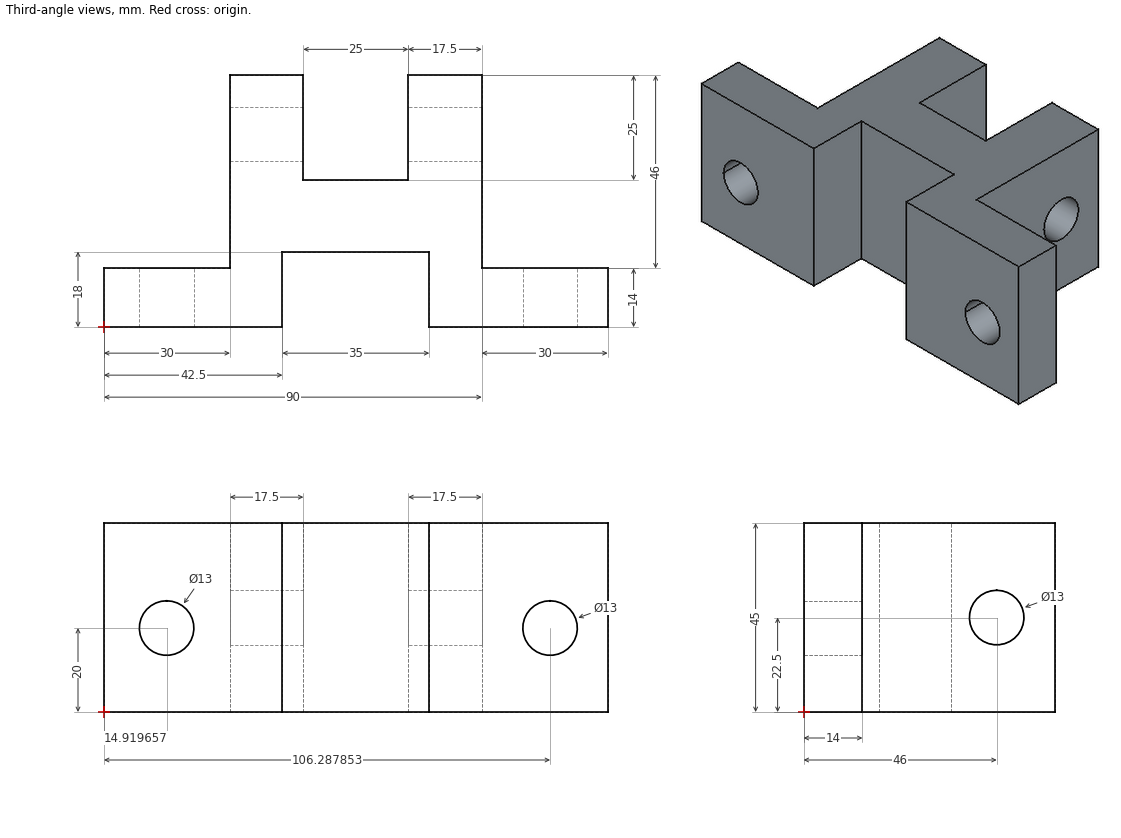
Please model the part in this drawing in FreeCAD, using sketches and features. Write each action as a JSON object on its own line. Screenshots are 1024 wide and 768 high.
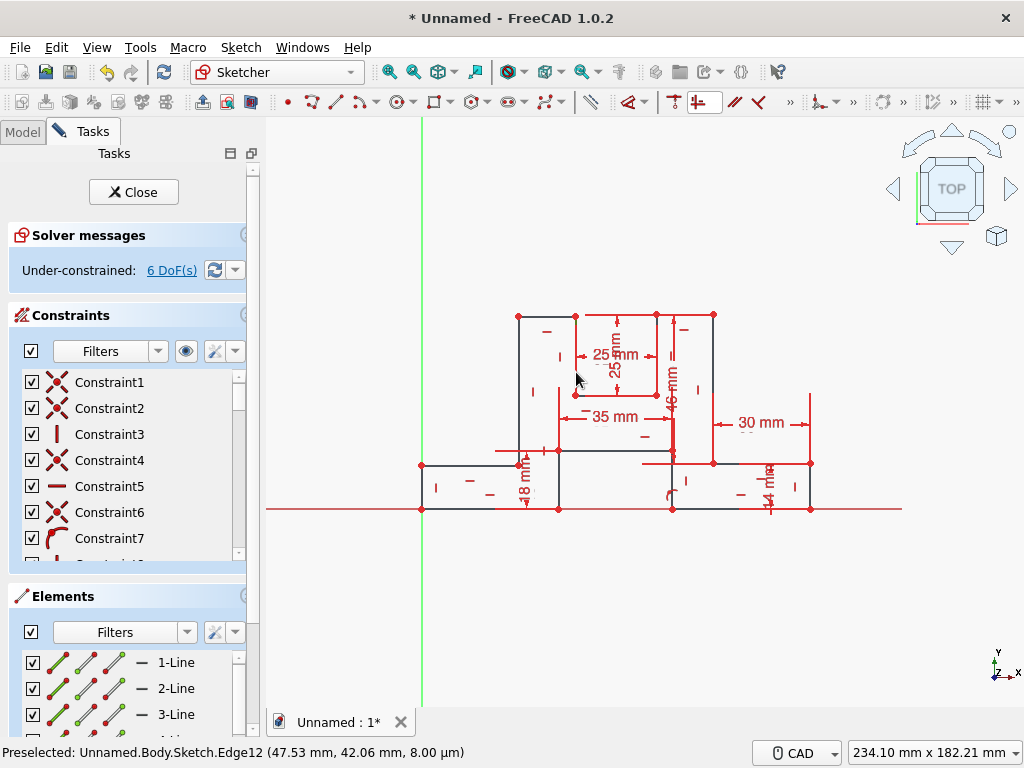
{"action": "key", "text": "i"}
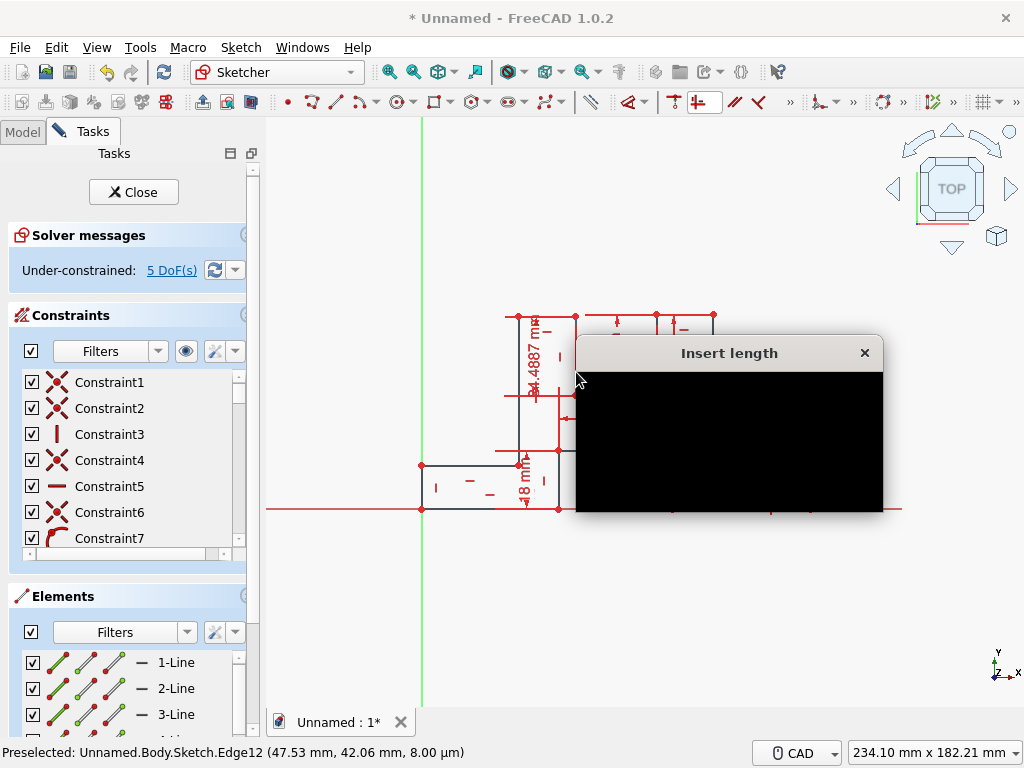
{"action": "type", "text": "25"}
{"action": "key", "text": "Return"}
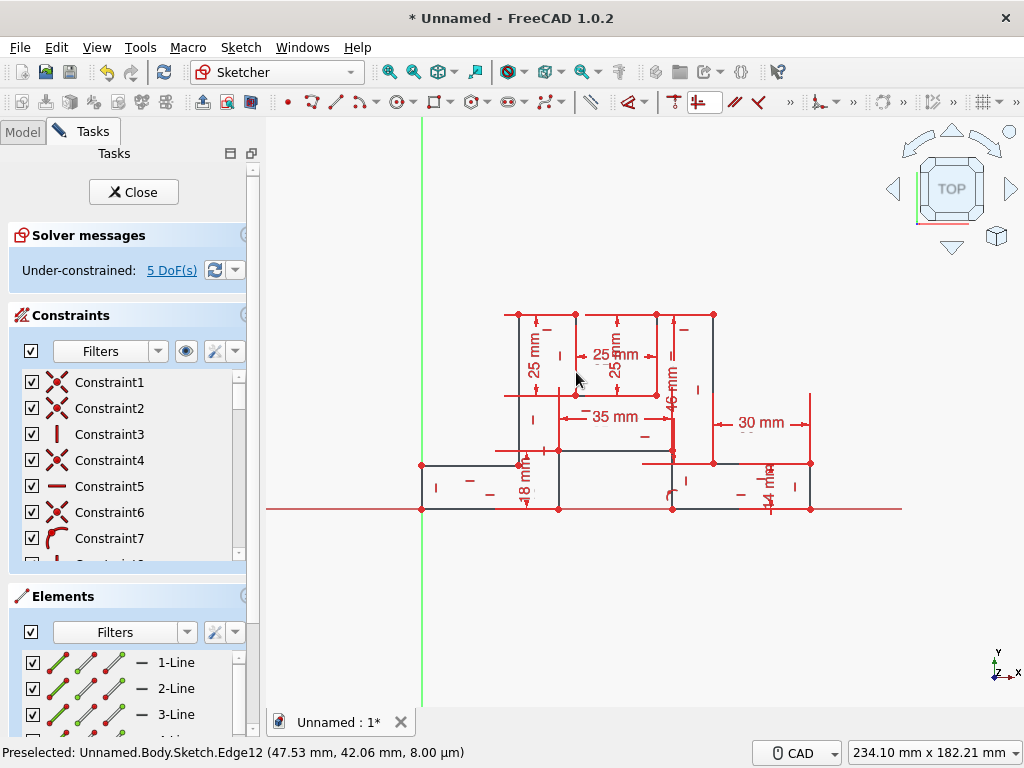
{"action": "left_click", "coordinate": [519, 360]}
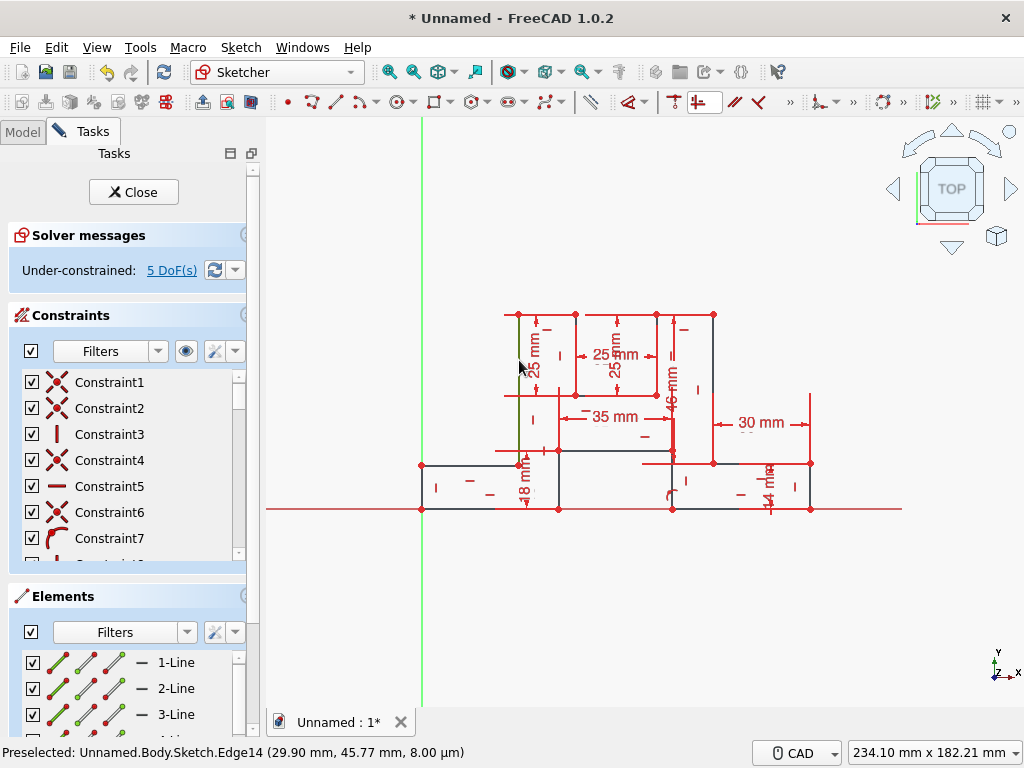
{"action": "left_click", "coordinate": [646, 102]}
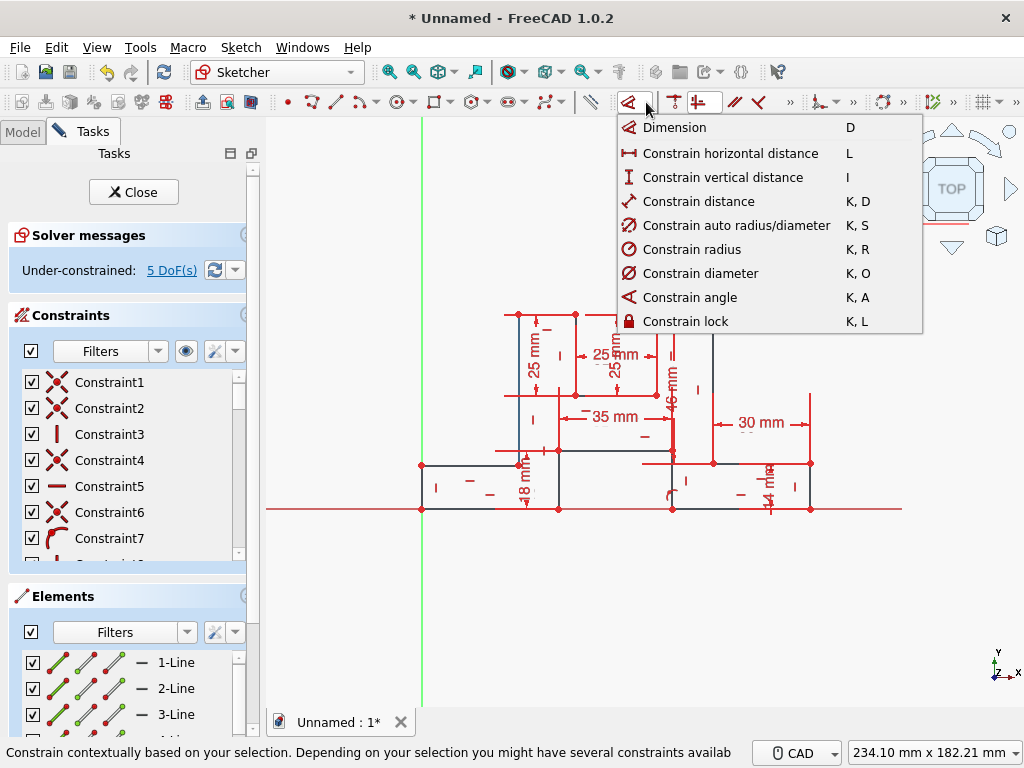
{"action": "left_click", "coordinate": [770, 177]}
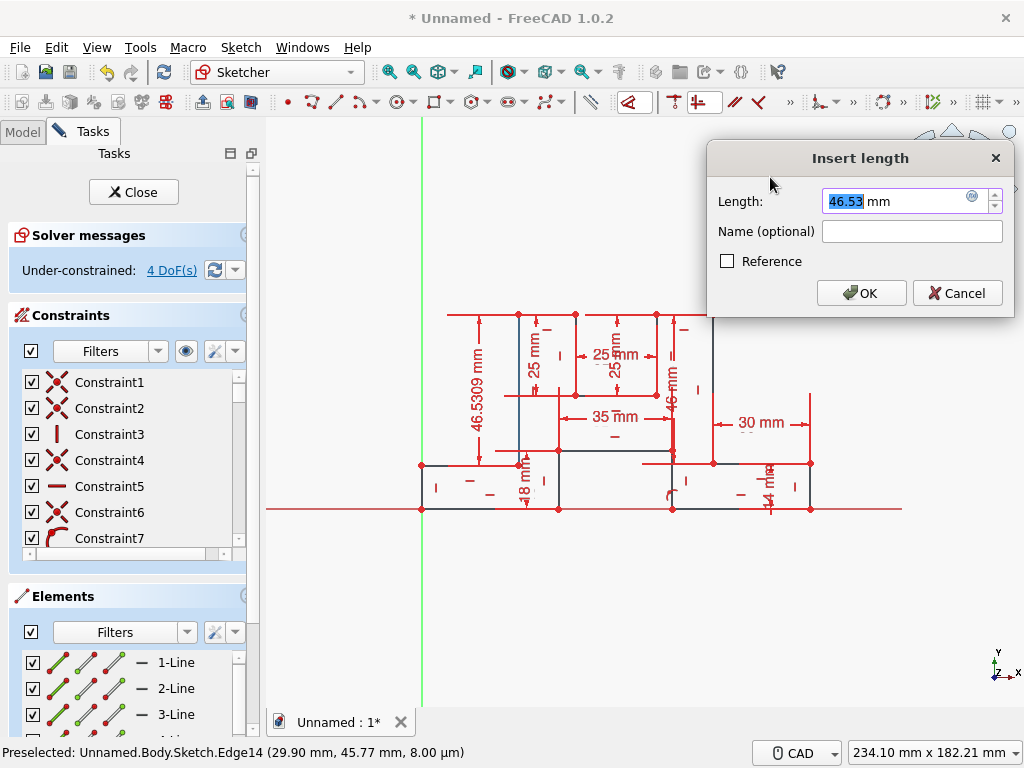
{"action": "type", "text": "46"}
{"action": "key", "text": "Return"}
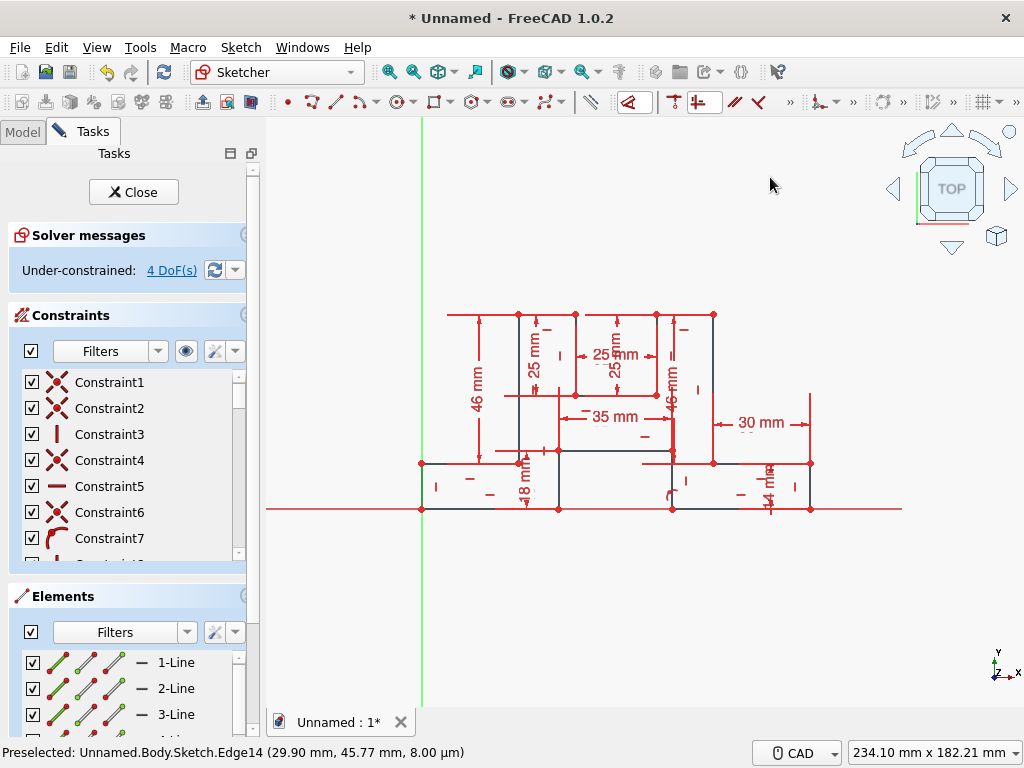
{"action": "left_click", "coordinate": [490, 464]}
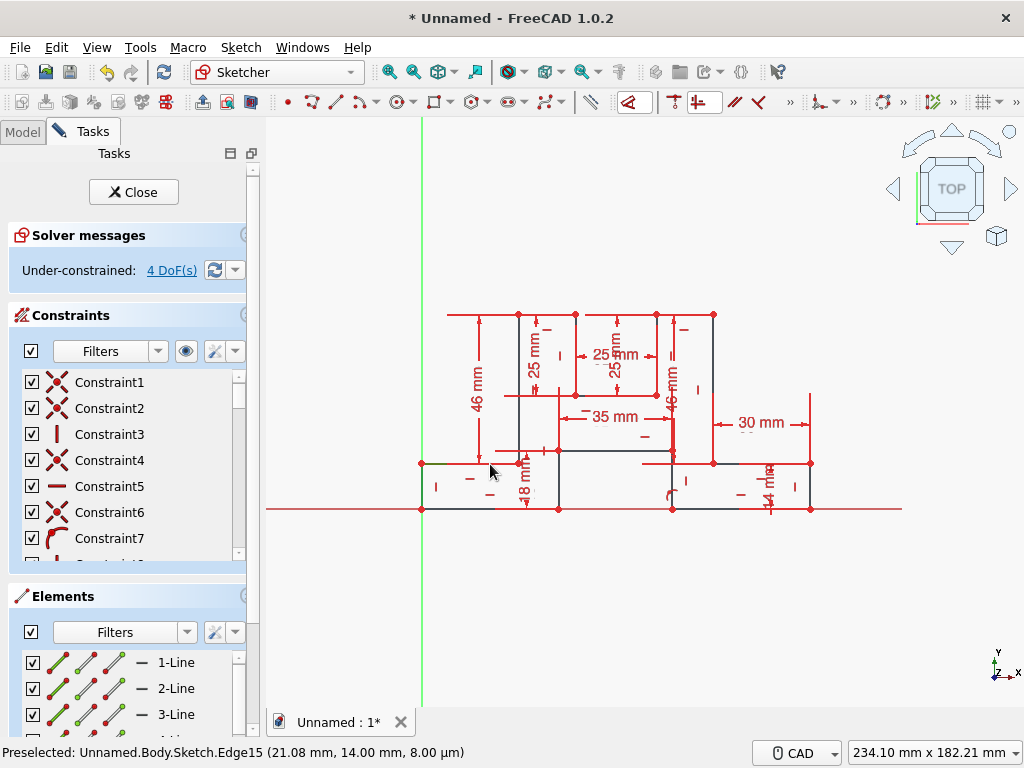
{"action": "key", "text": "l"}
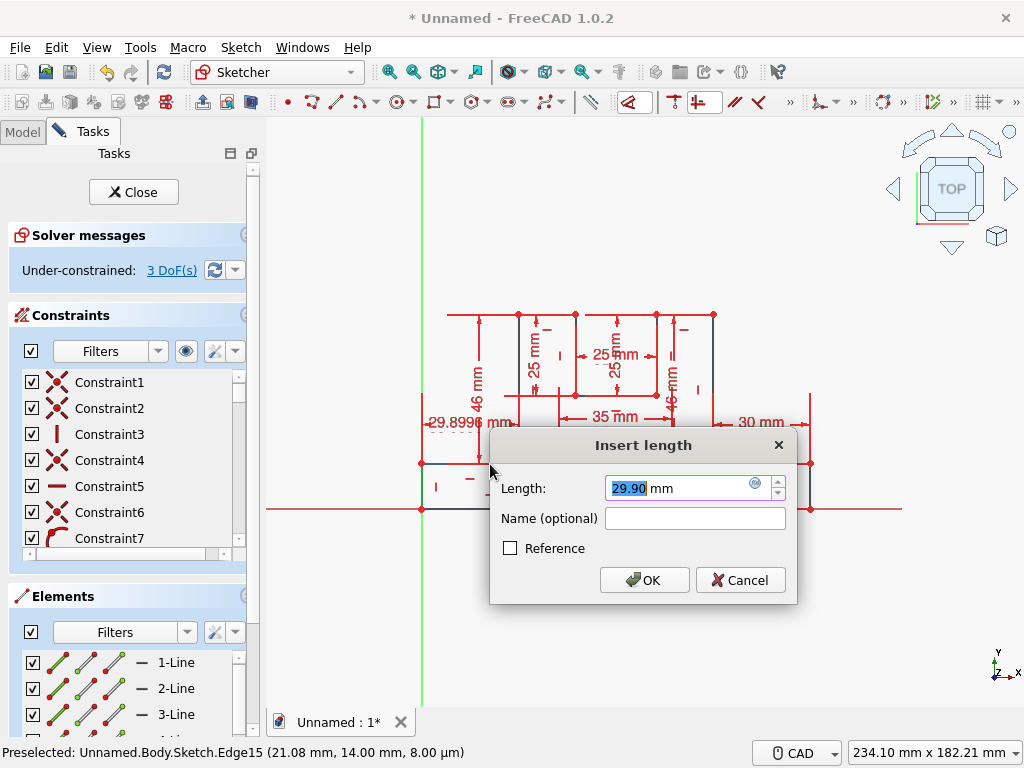
{"action": "type", "text": "30"}
{"action": "key", "text": "Return"}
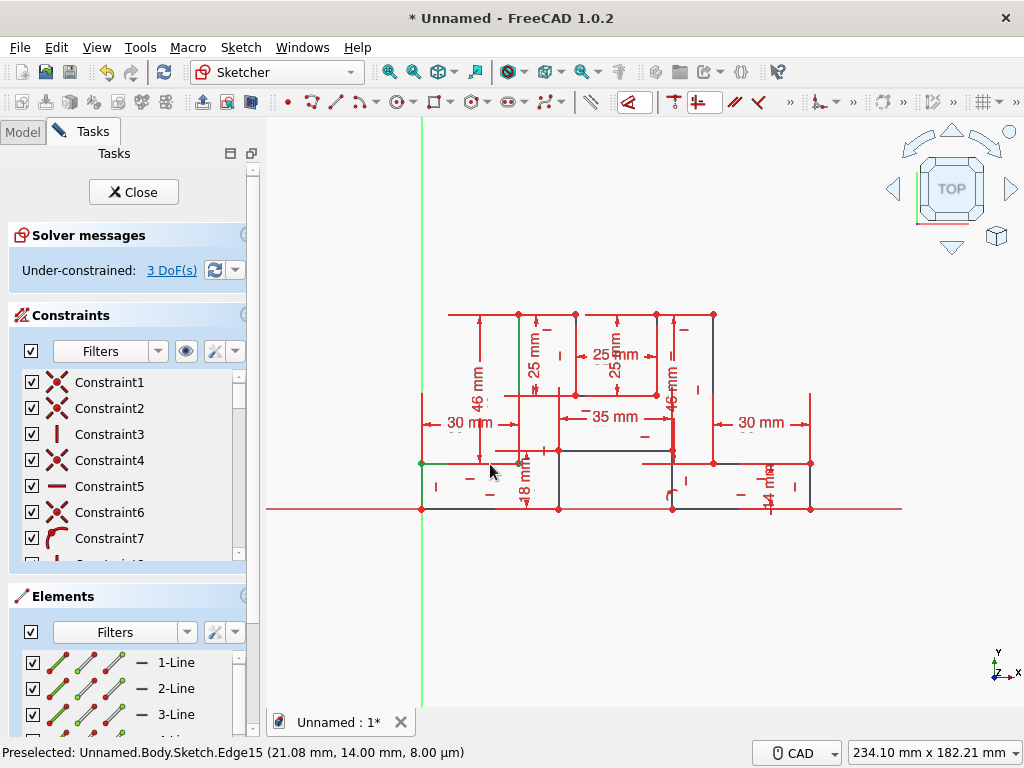
{"action": "left_click", "coordinate": [713, 464]}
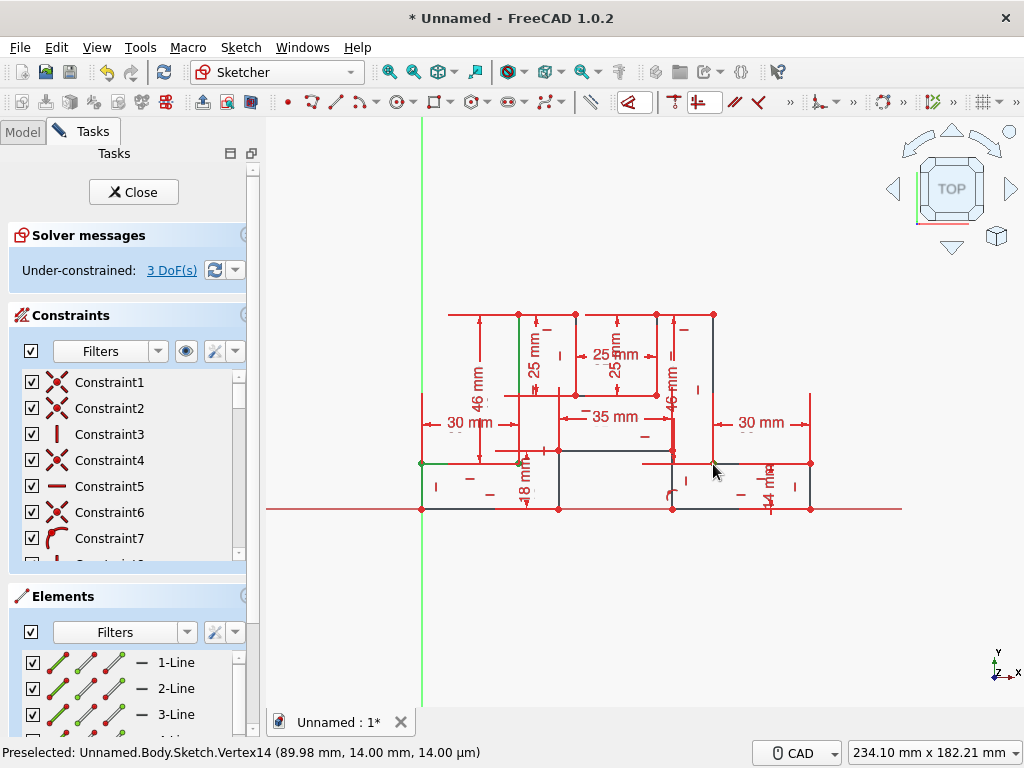
{"action": "key", "text": "l"}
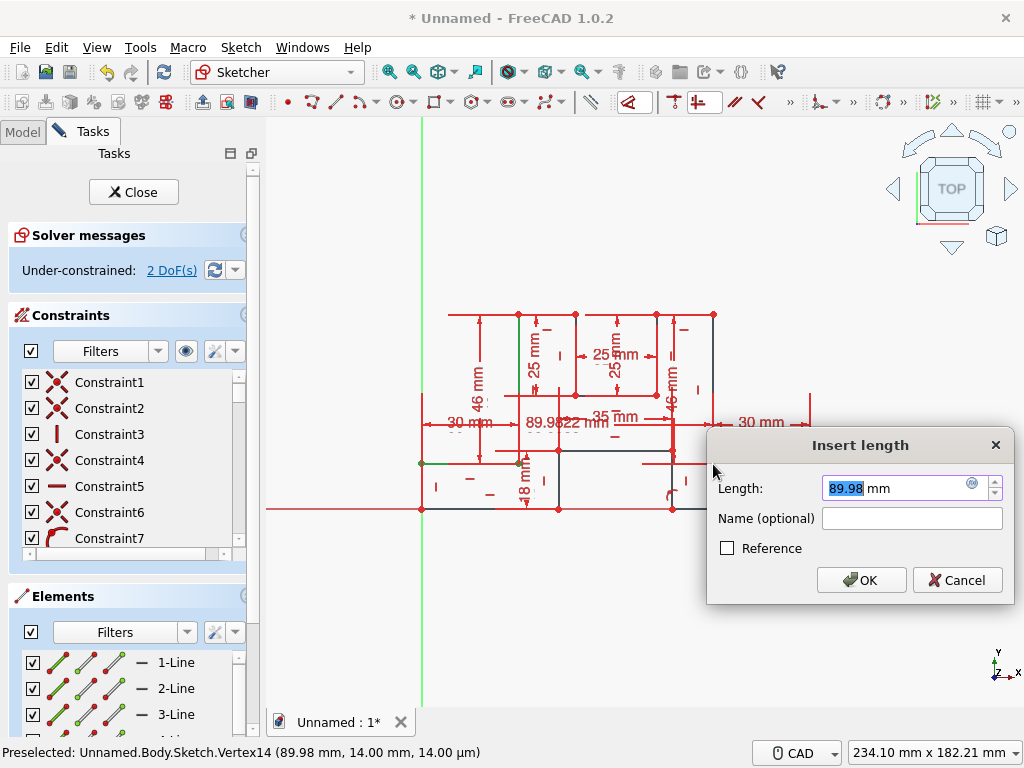
{"action": "type", "text": "90"}
{"action": "key", "text": "Return"}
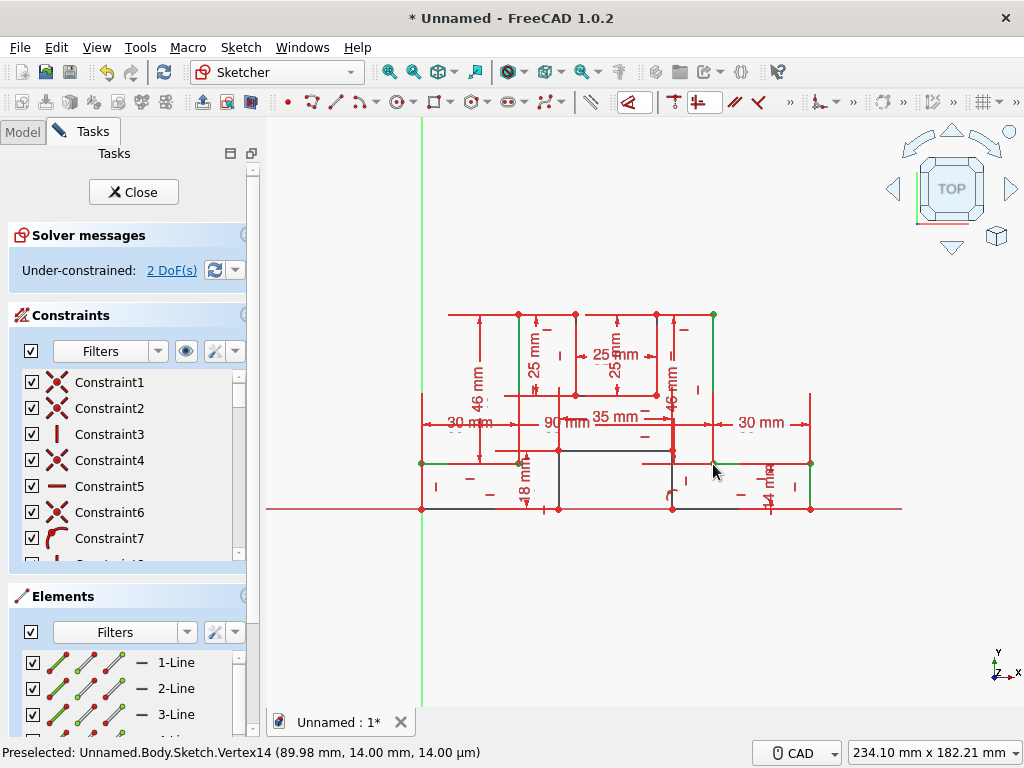
{"action": "left_click", "coordinate": [463, 509]}